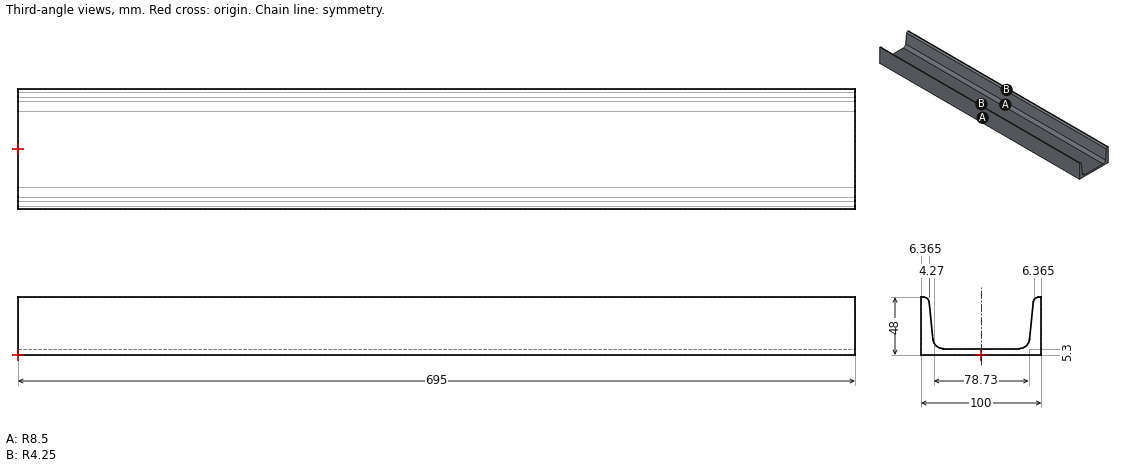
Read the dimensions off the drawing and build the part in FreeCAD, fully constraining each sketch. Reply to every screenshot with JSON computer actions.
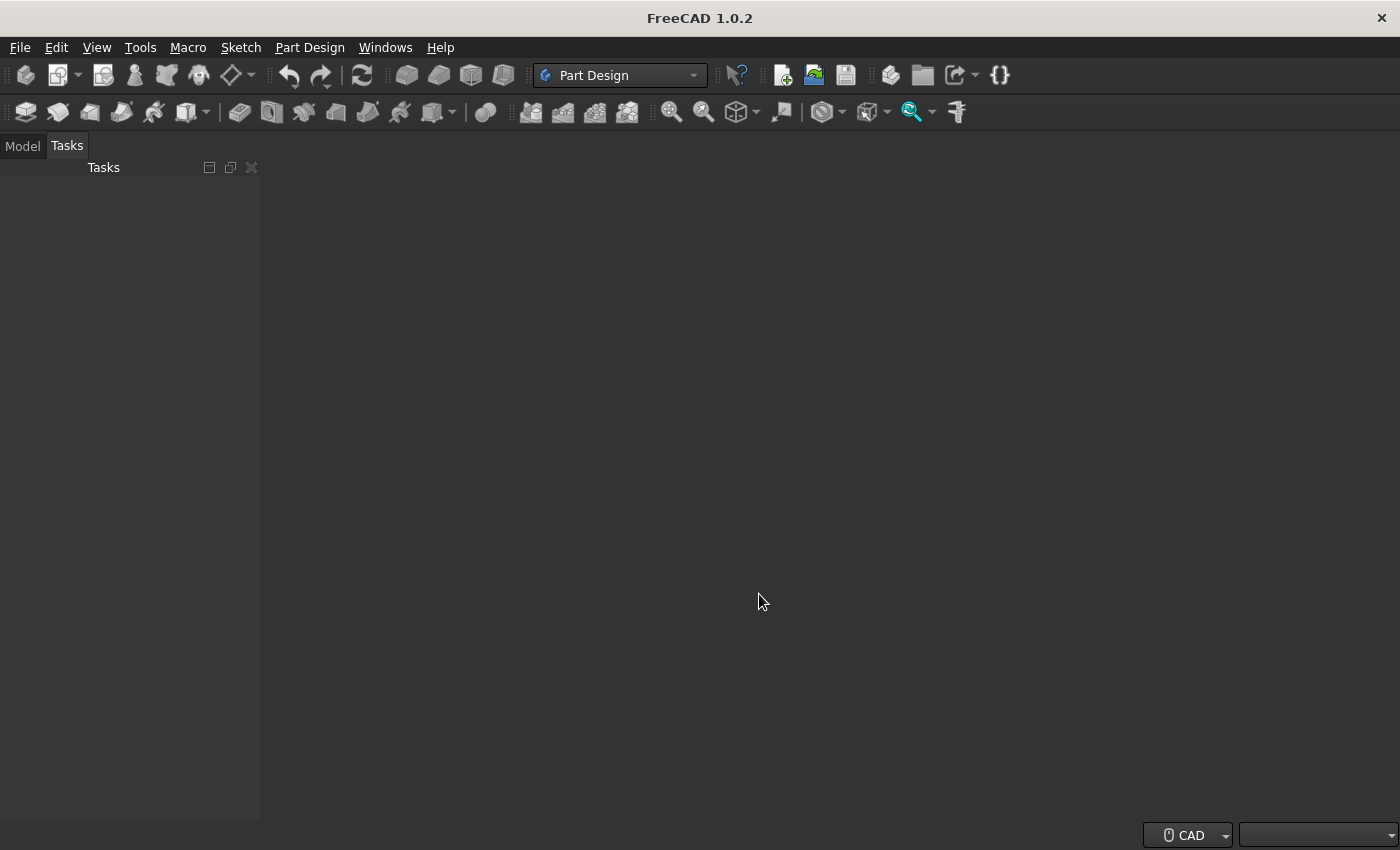
{"action": "left_click", "coordinate": [782, 76]}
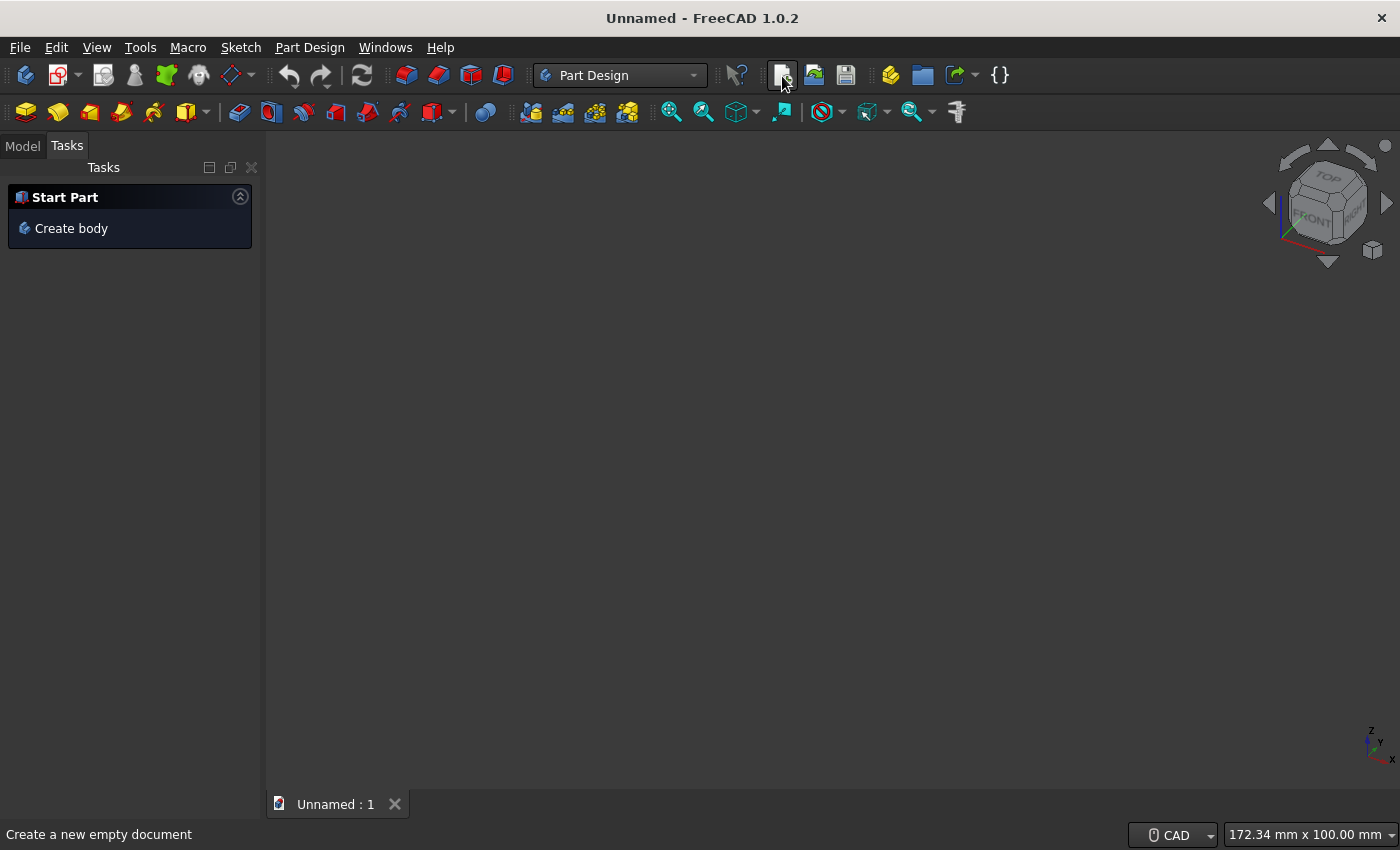
{"action": "left_click", "coordinate": [58, 76]}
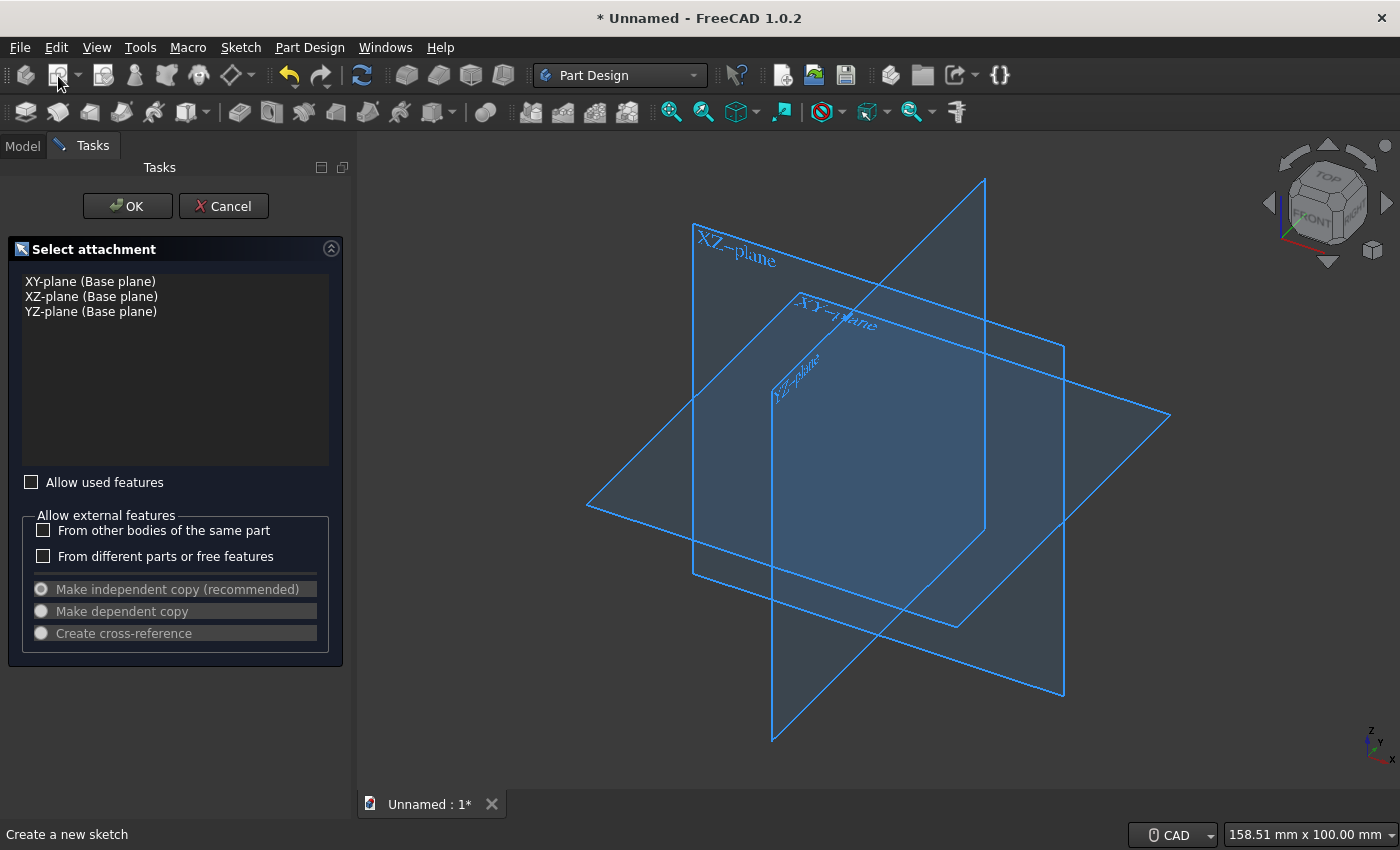
{"action": "left_click", "coordinate": [82, 312]}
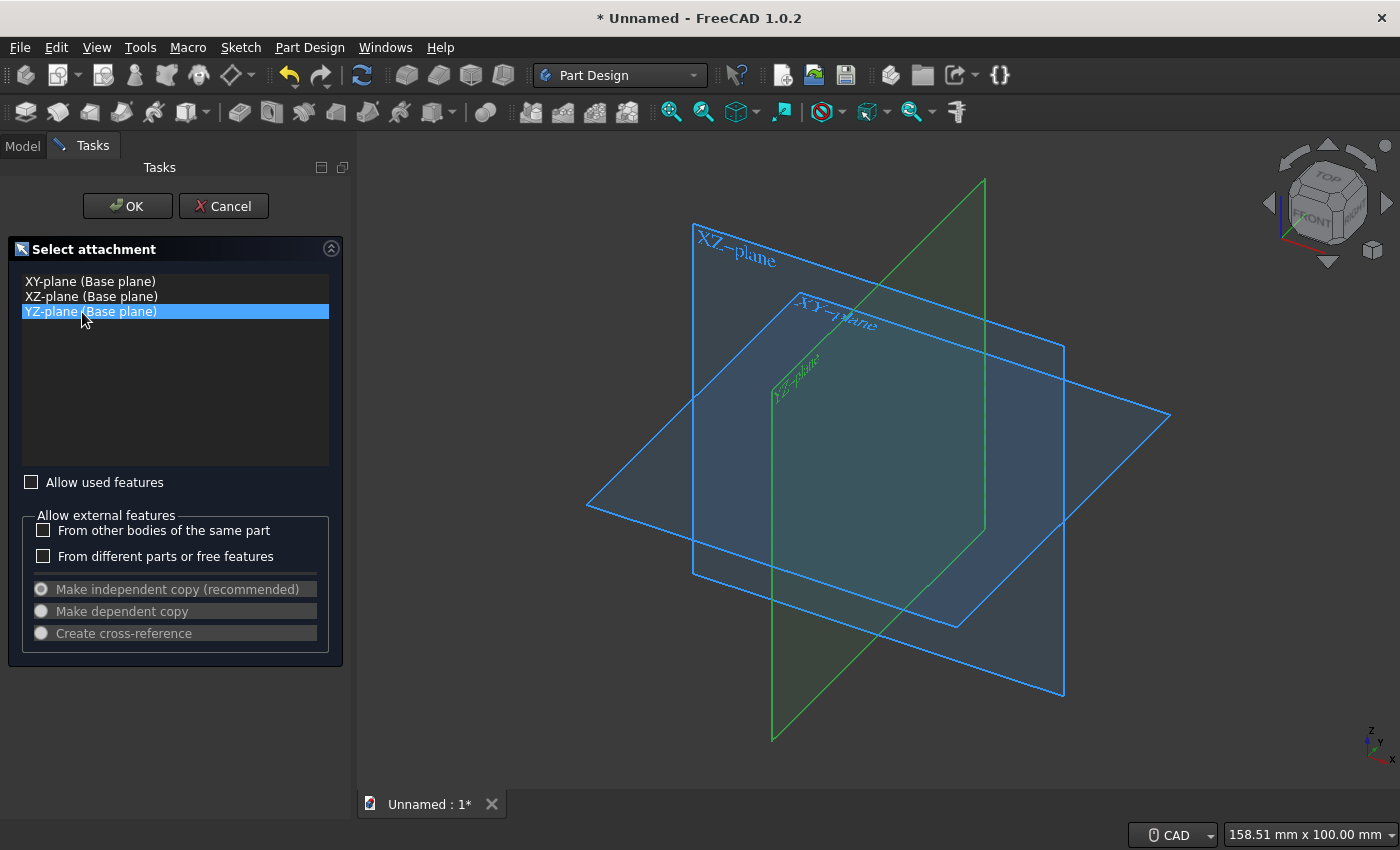
{"action": "left_click", "coordinate": [128, 206]}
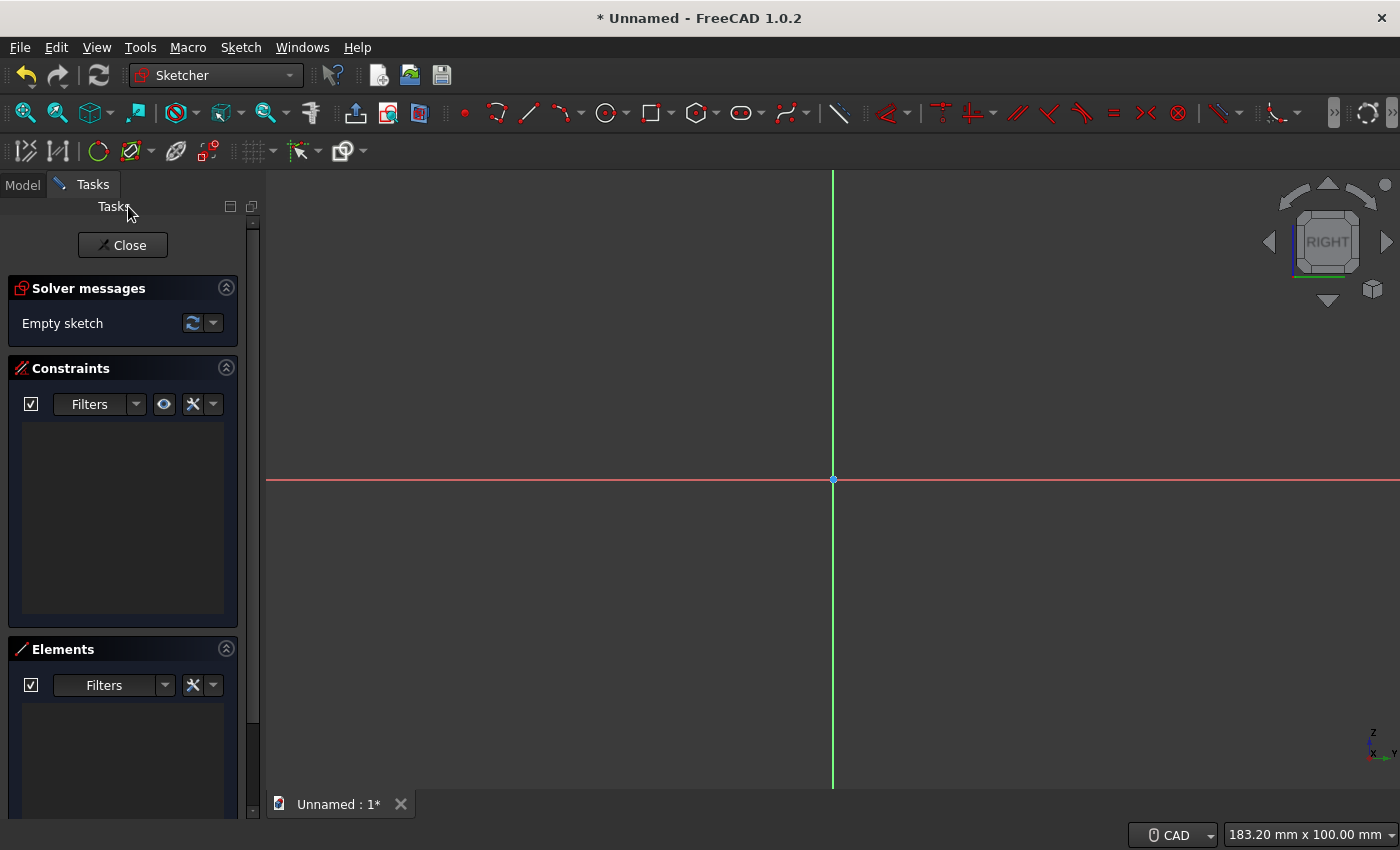
{"action": "scroll", "coordinate": [455, 761], "scroll_direction": "down", "scroll_amount": 1}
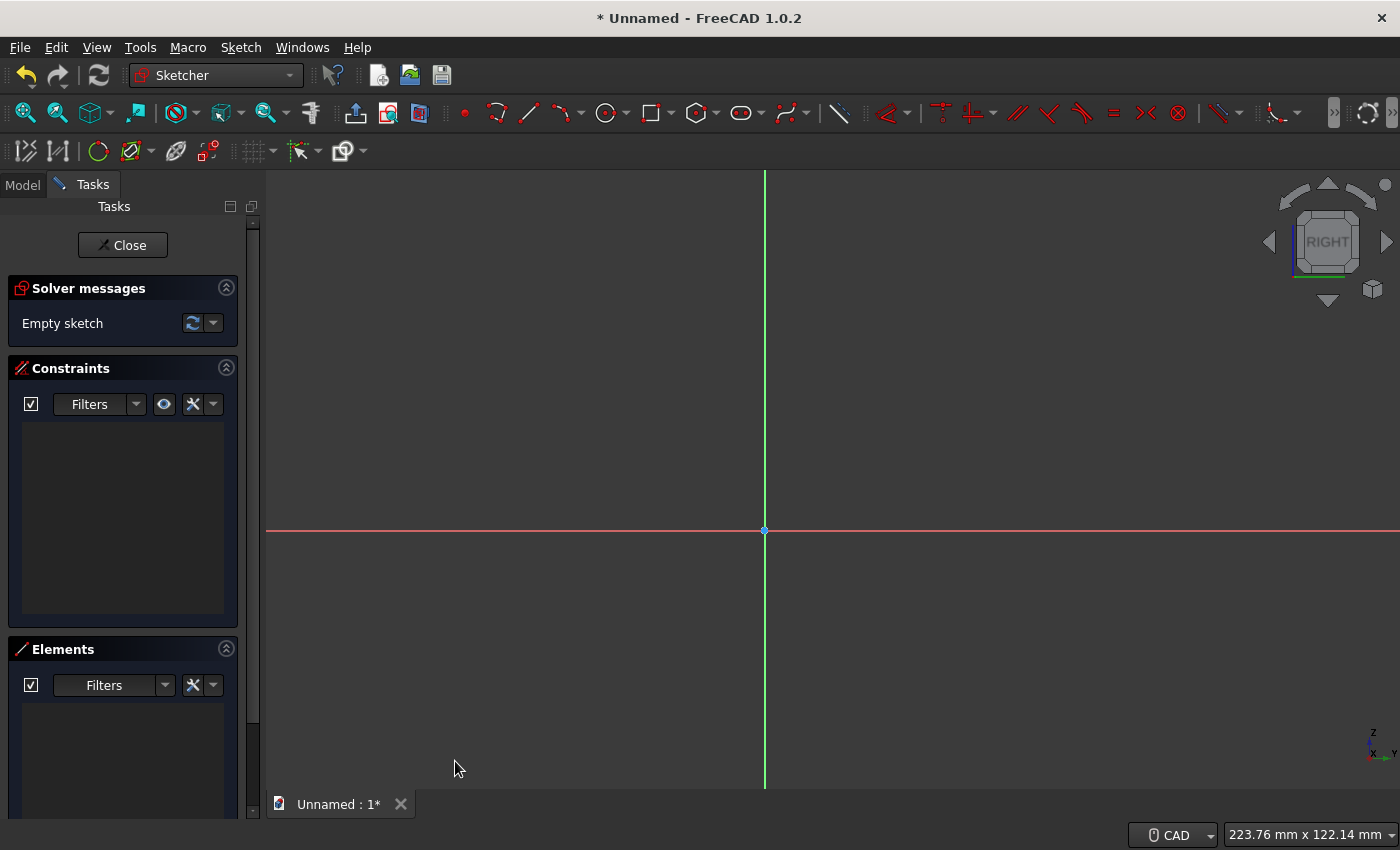
{"action": "left_click", "coordinate": [498, 114]}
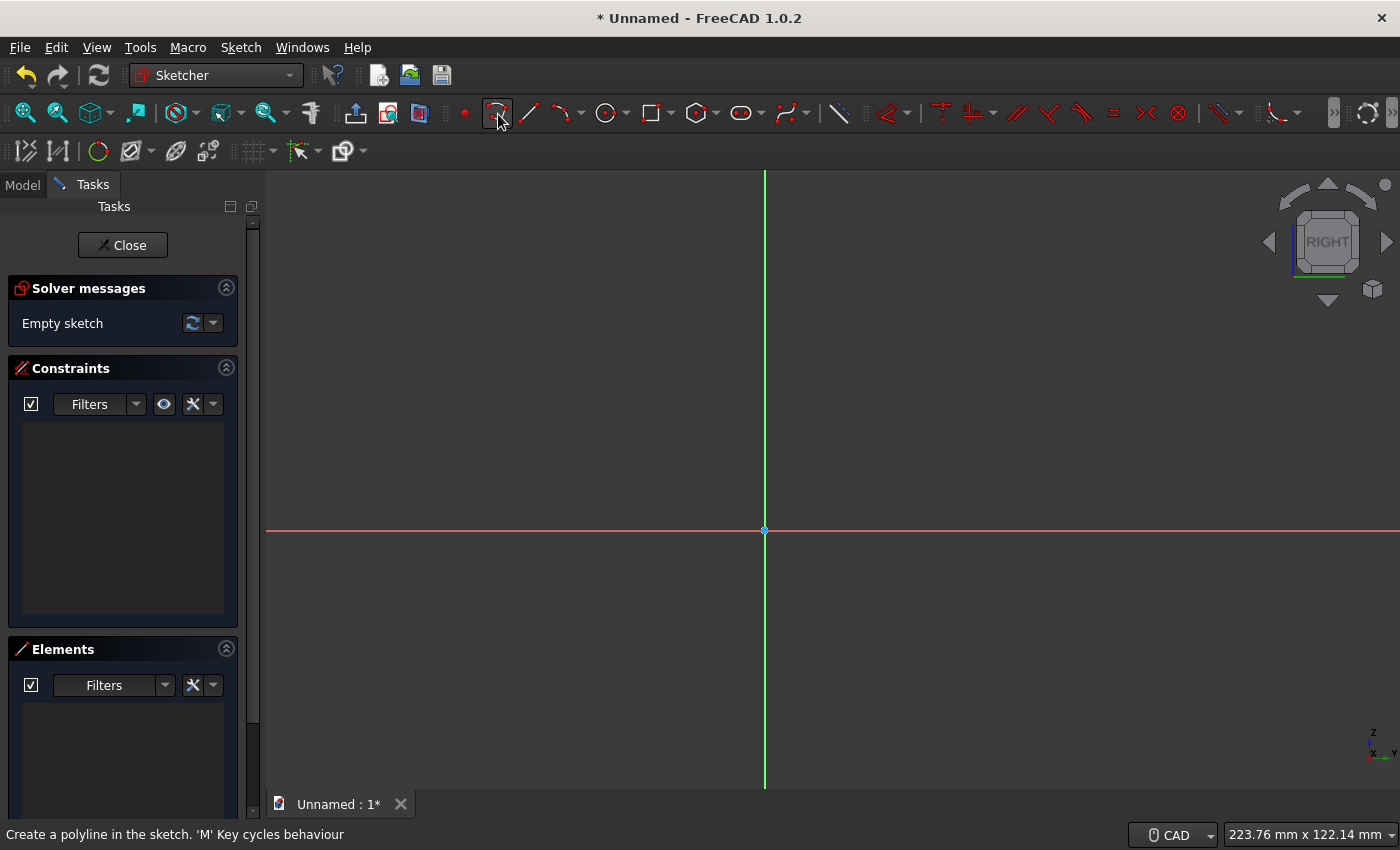
{"action": "left_click", "coordinate": [964, 504]}
{"action": "left_click", "coordinate": [565, 504]}
{"action": "left_click", "coordinate": [543, 287]}
{"action": "left_click", "coordinate": [511, 287]}
{"action": "left_click", "coordinate": [511, 531]}
{"action": "left_click", "coordinate": [1018, 522]}
{"action": "left_click", "coordinate": [1018, 287]}
{"action": "left_click", "coordinate": [986, 287]}
{"action": "left_click", "coordinate": [964, 505]}
{"action": "key", "text": "Escape"}
{"action": "key", "text": "Escape"}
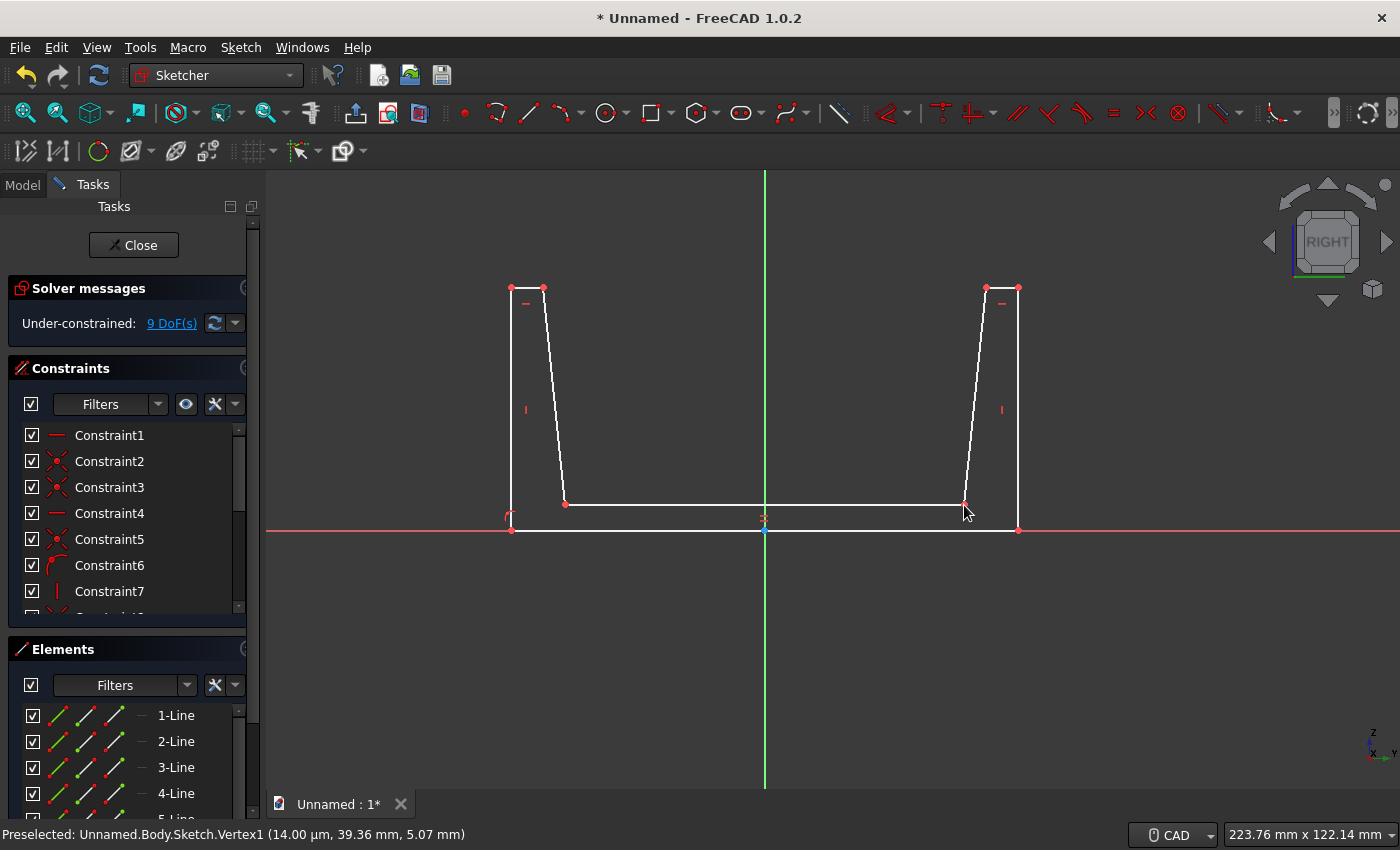
{"action": "left_click", "coordinate": [511, 288]}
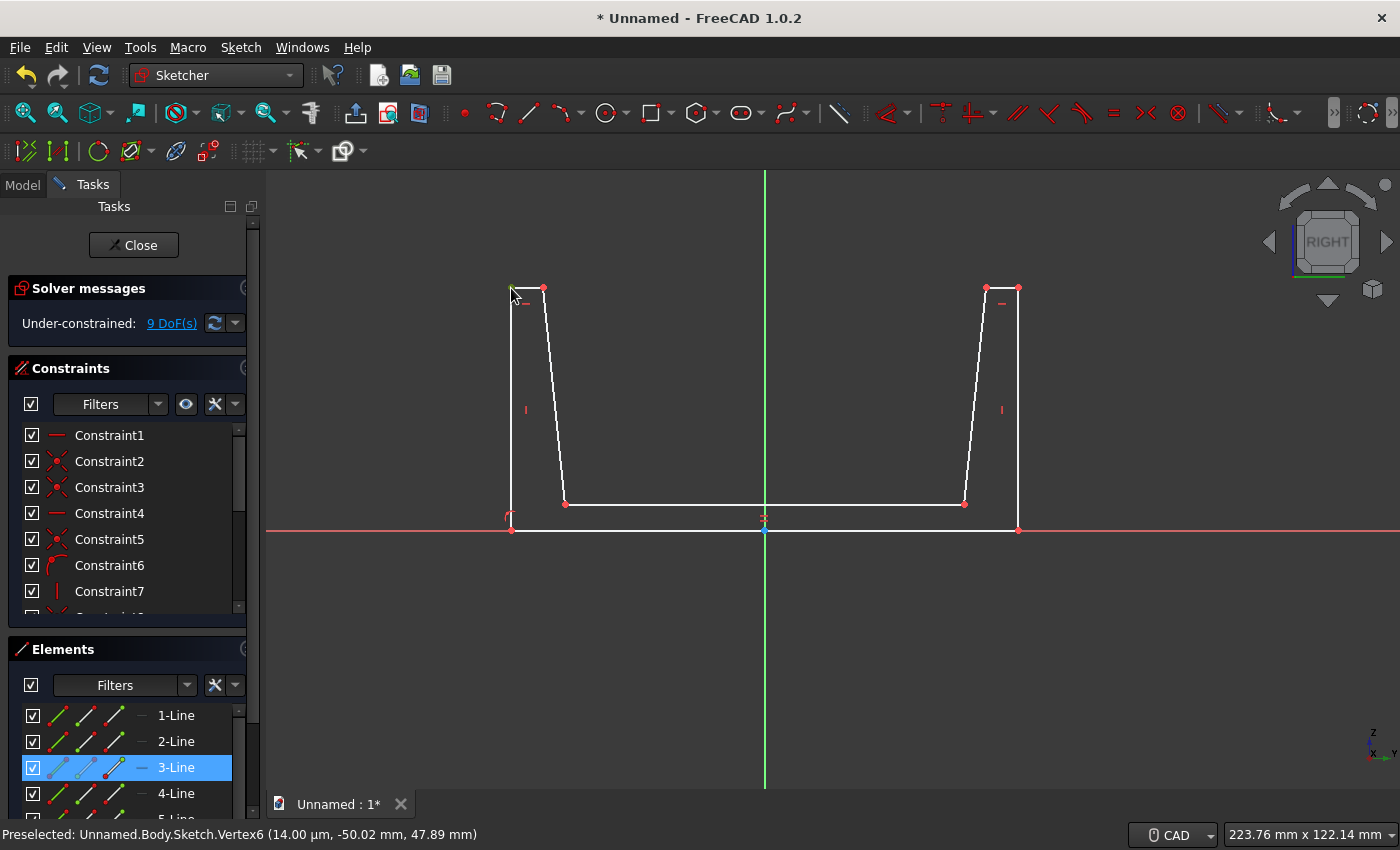
{"action": "left_click", "coordinate": [1018, 288]}